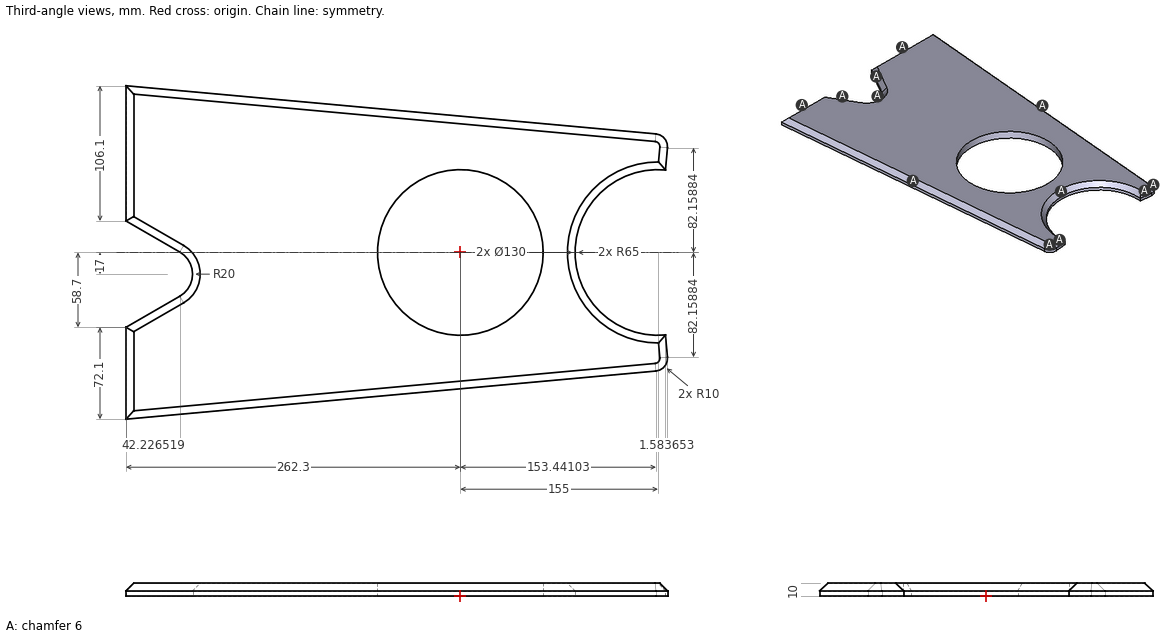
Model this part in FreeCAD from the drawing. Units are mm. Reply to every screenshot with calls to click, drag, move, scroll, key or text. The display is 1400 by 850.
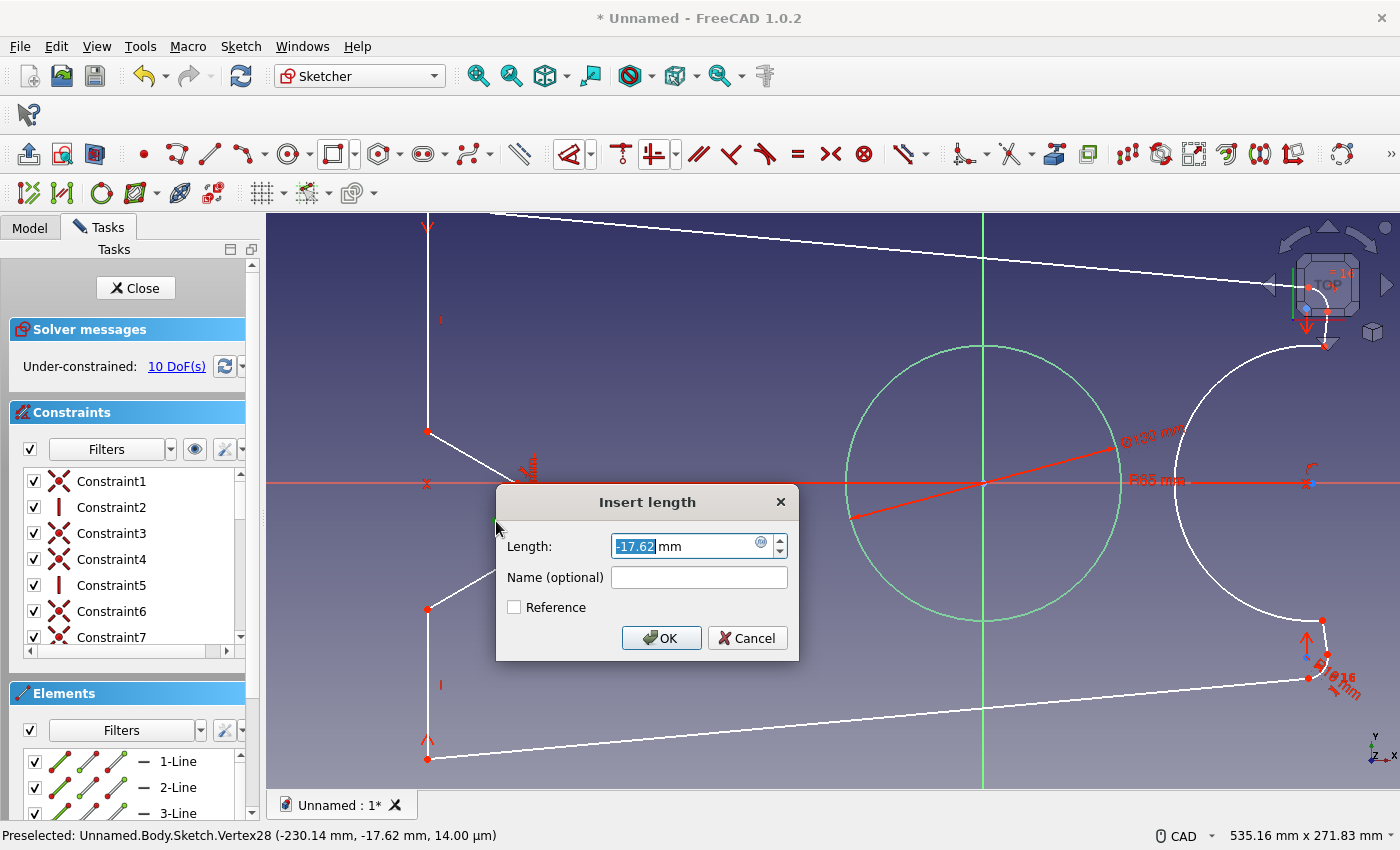
text(-17)
key(Return)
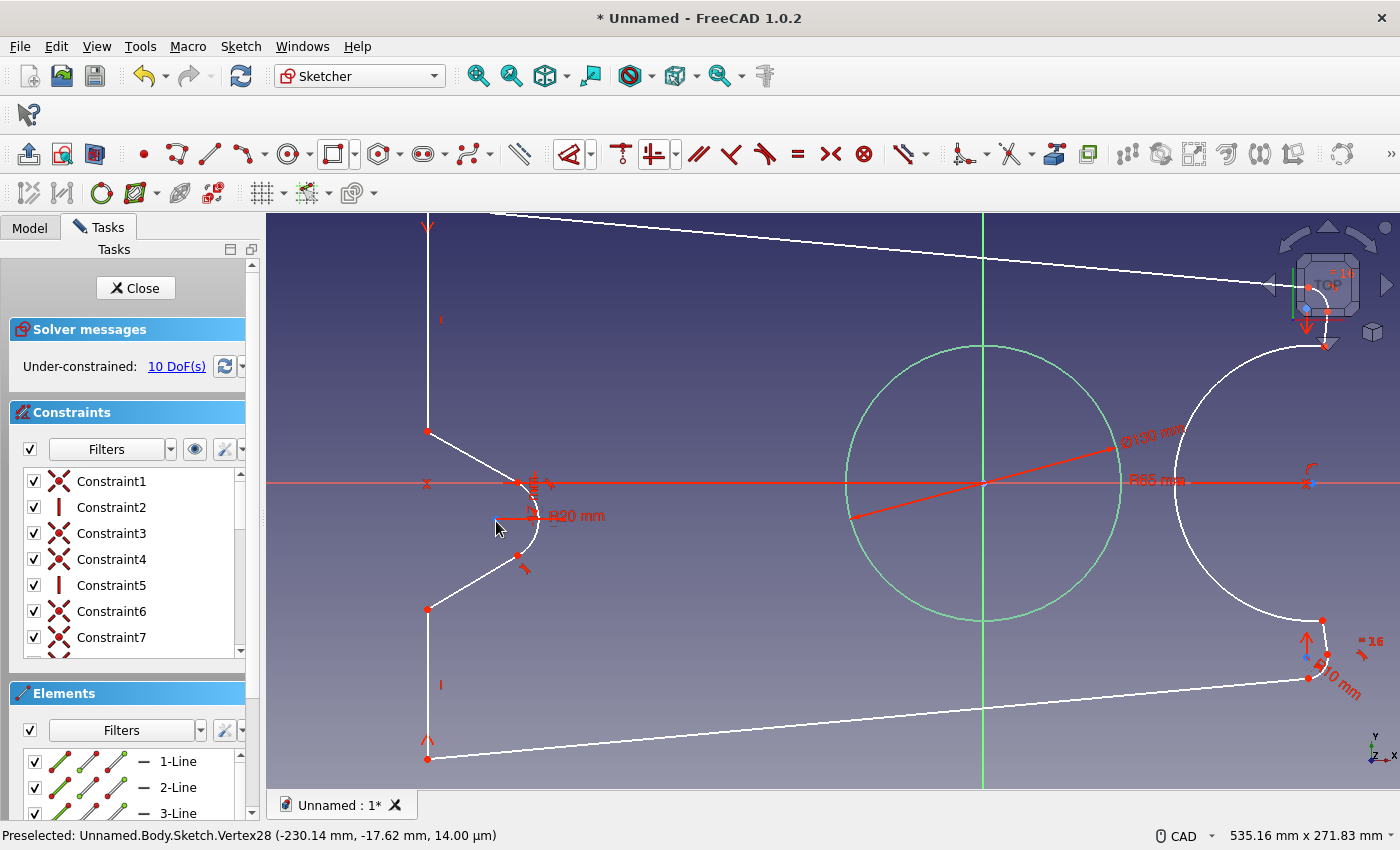
click(428, 654)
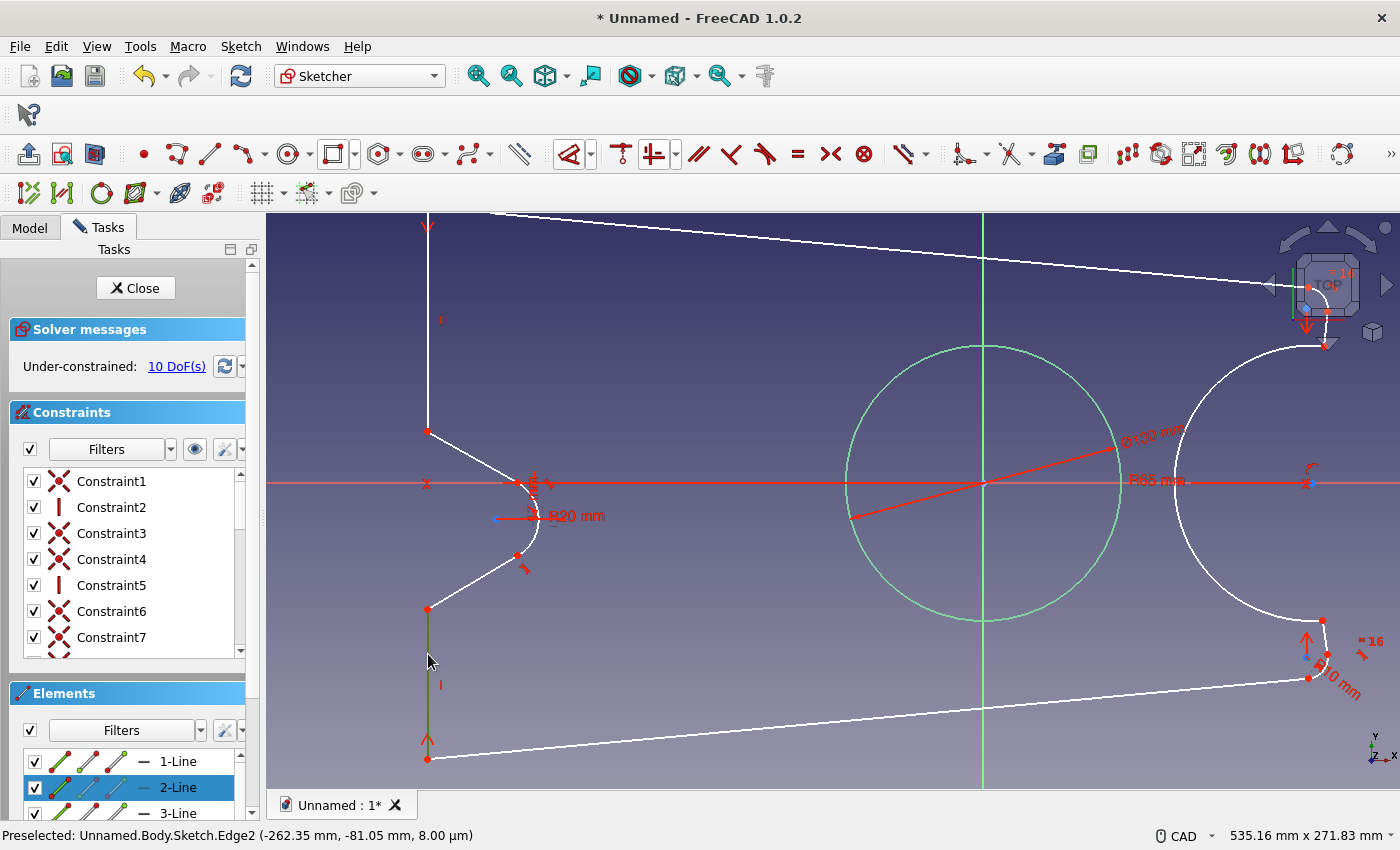
key(i)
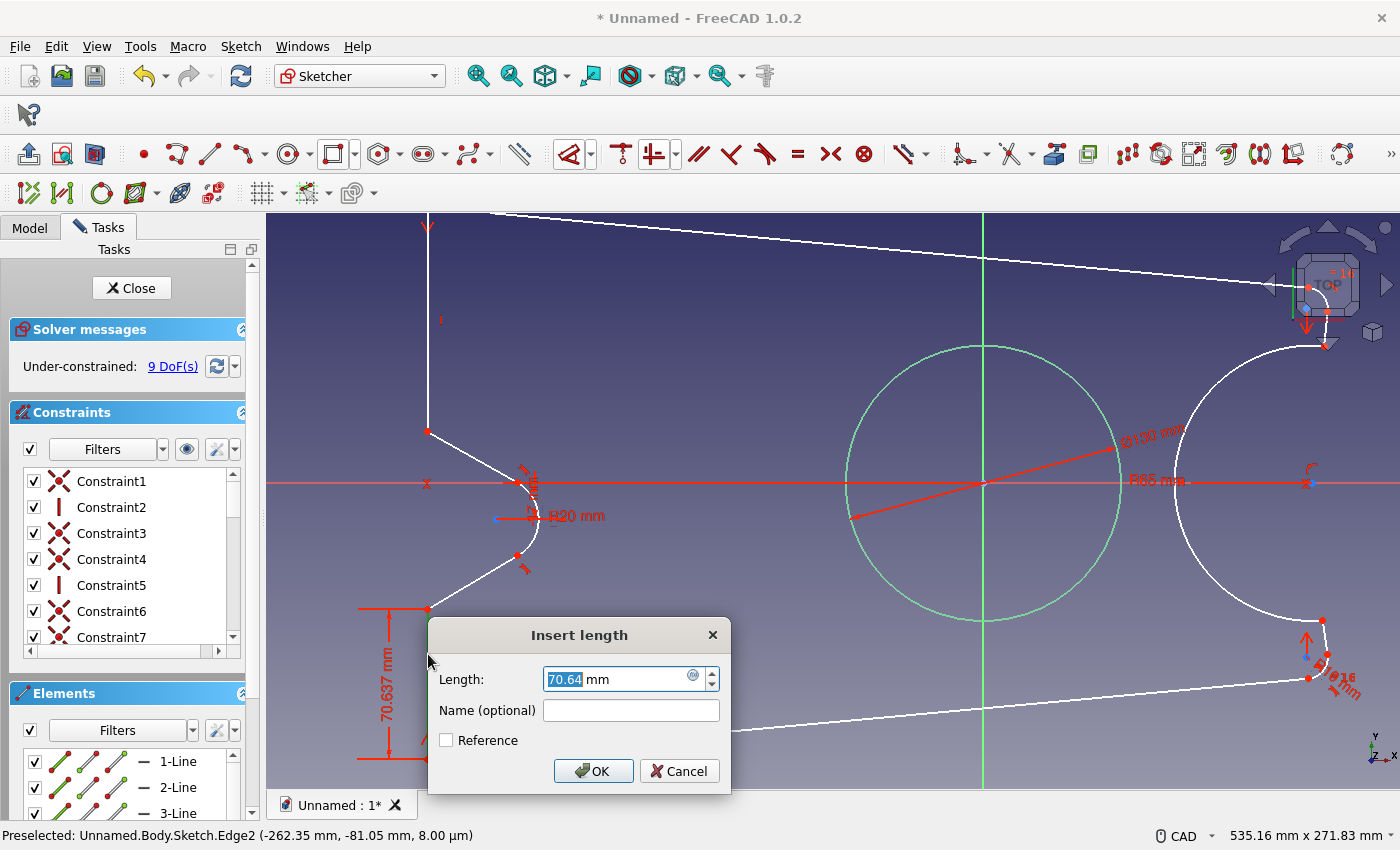
text(72.1)
key(Return)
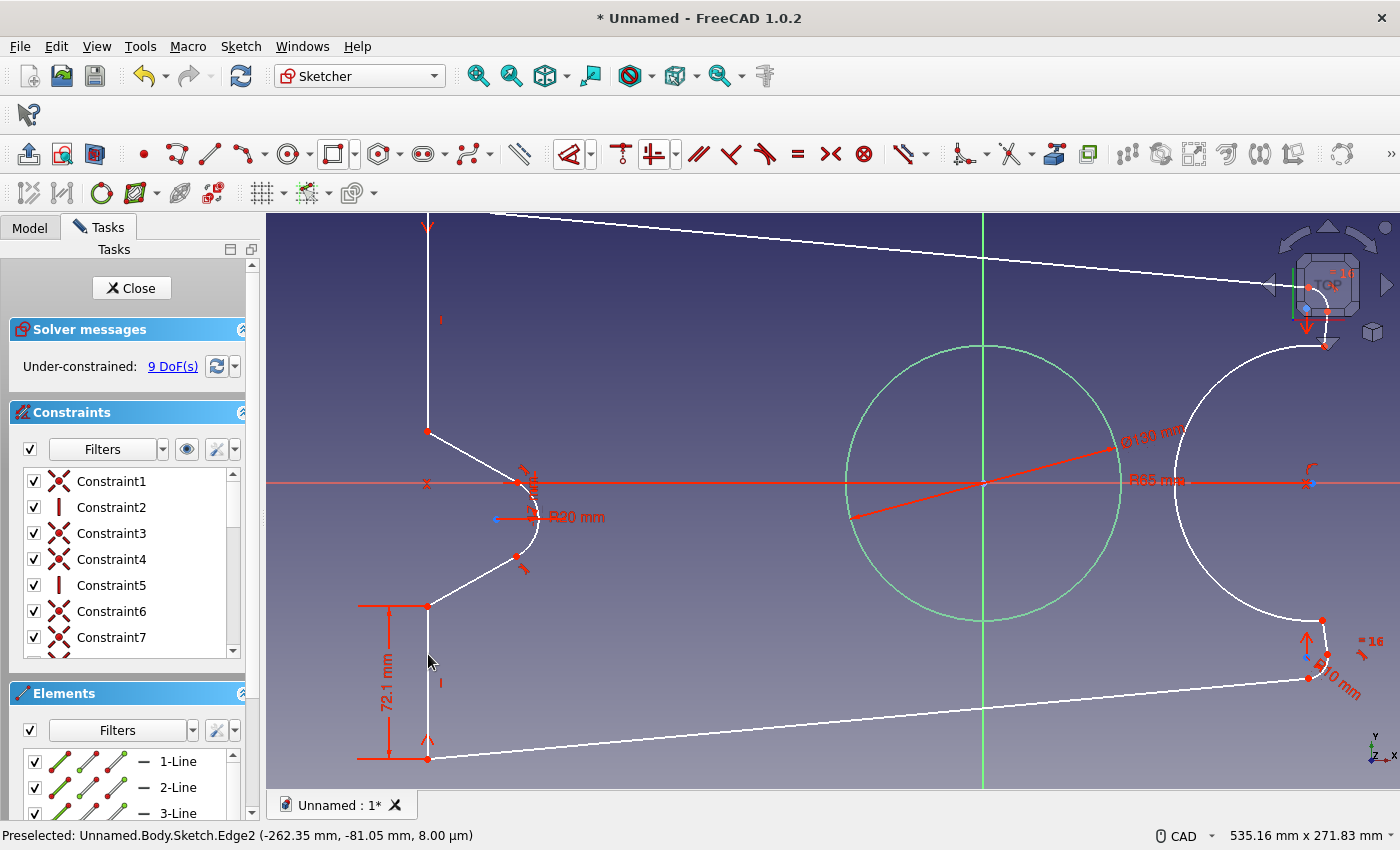
scroll(534, 537, down, 2)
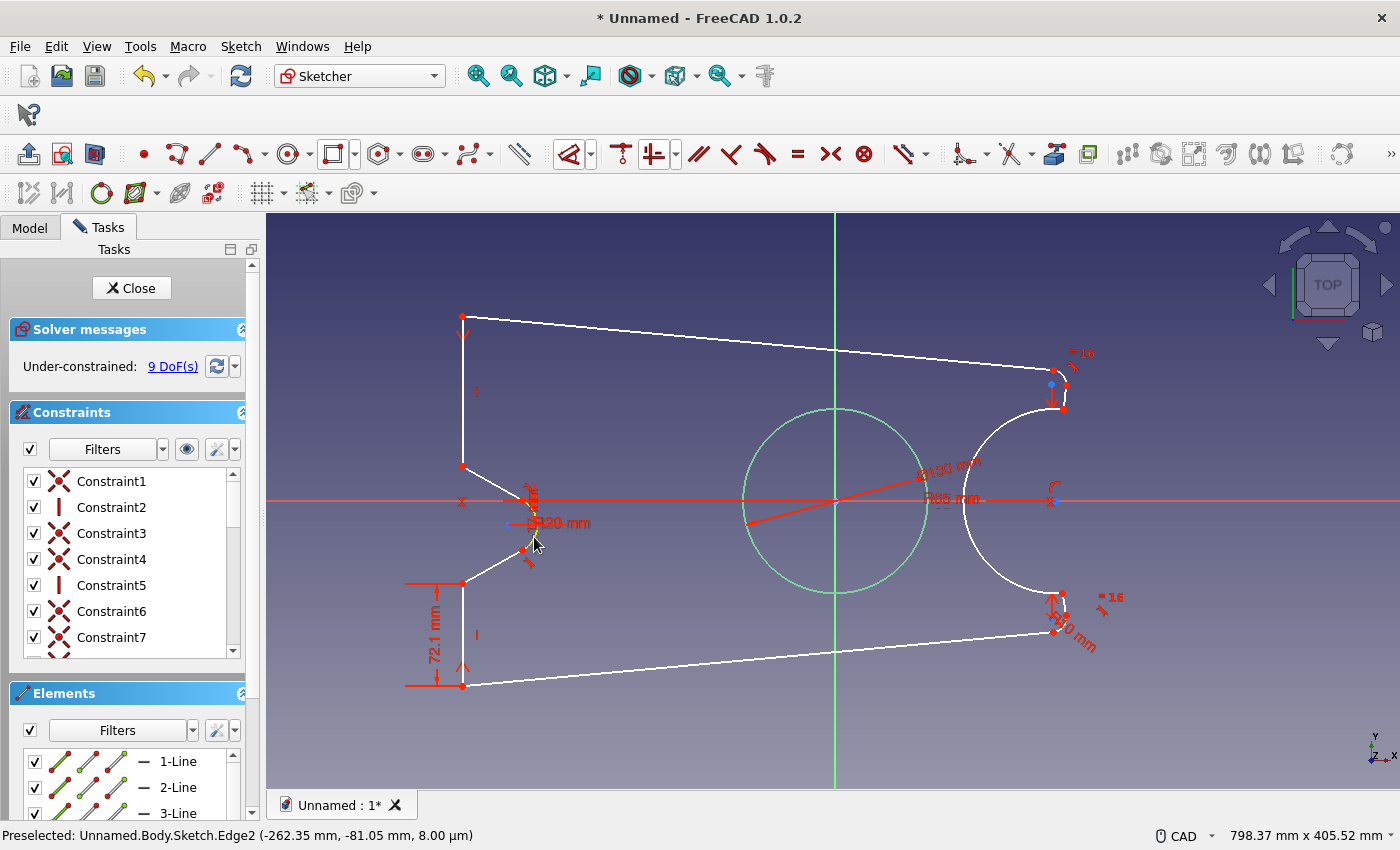
click(1056, 501)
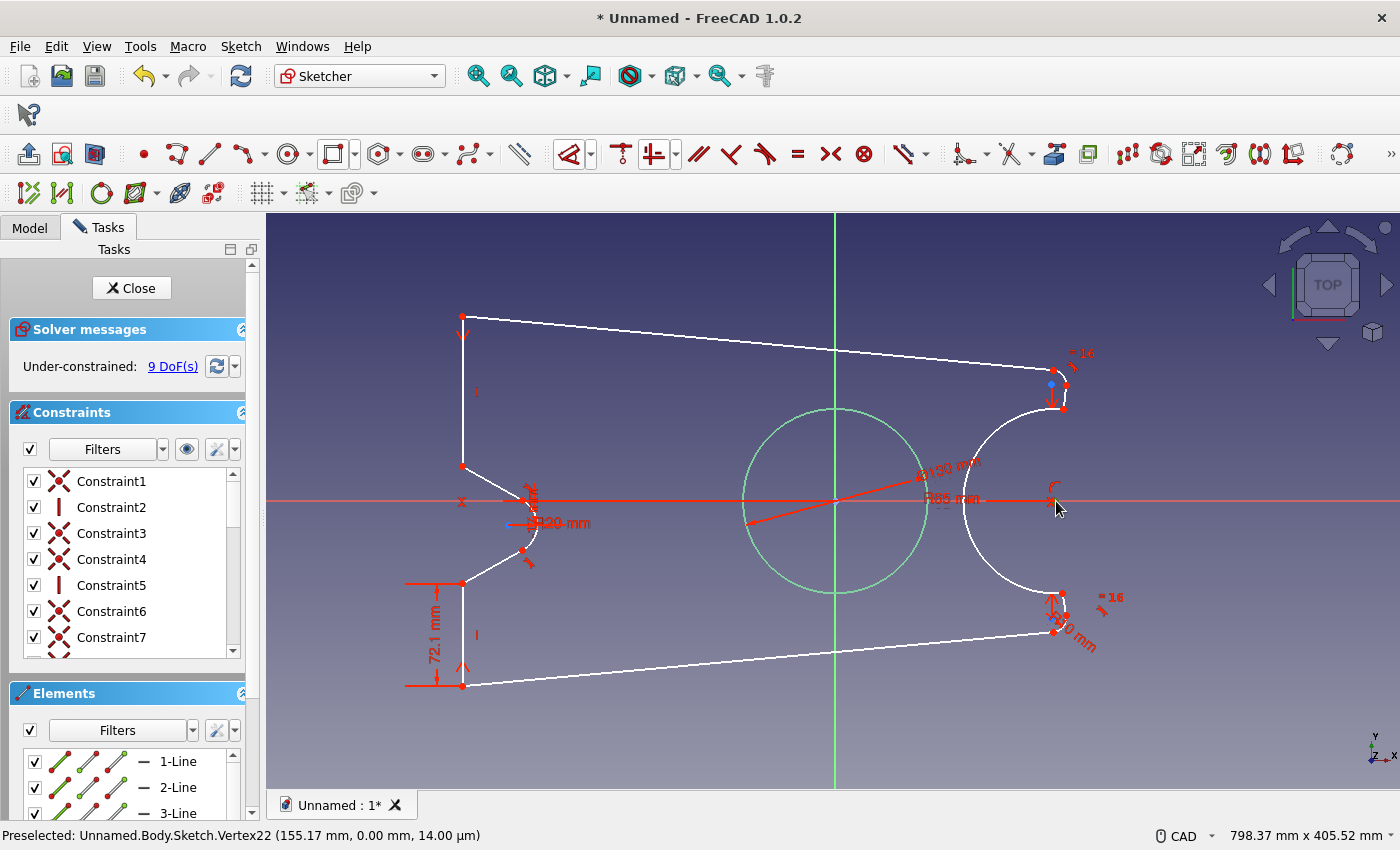
key(l)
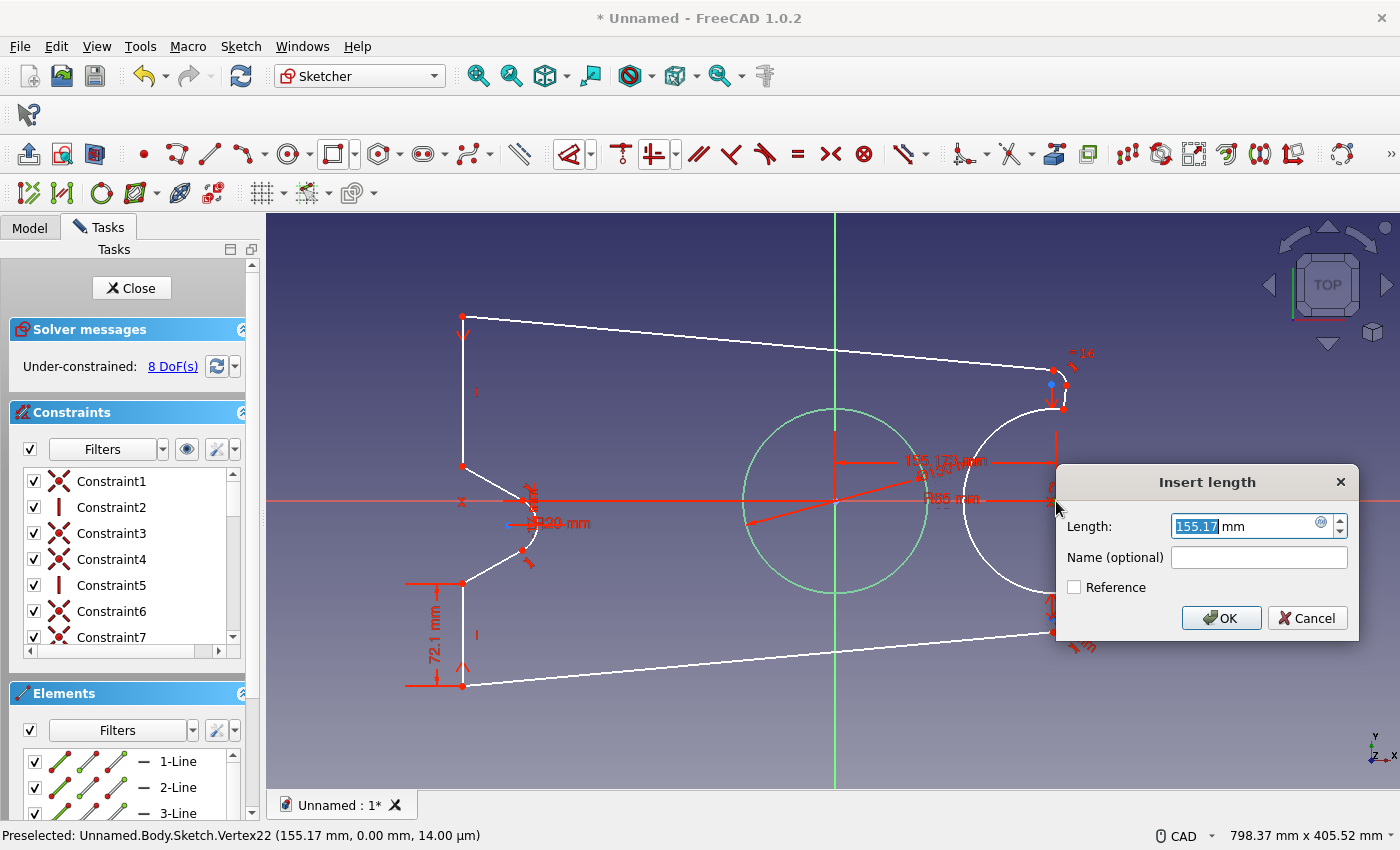
text(155)
key(Return)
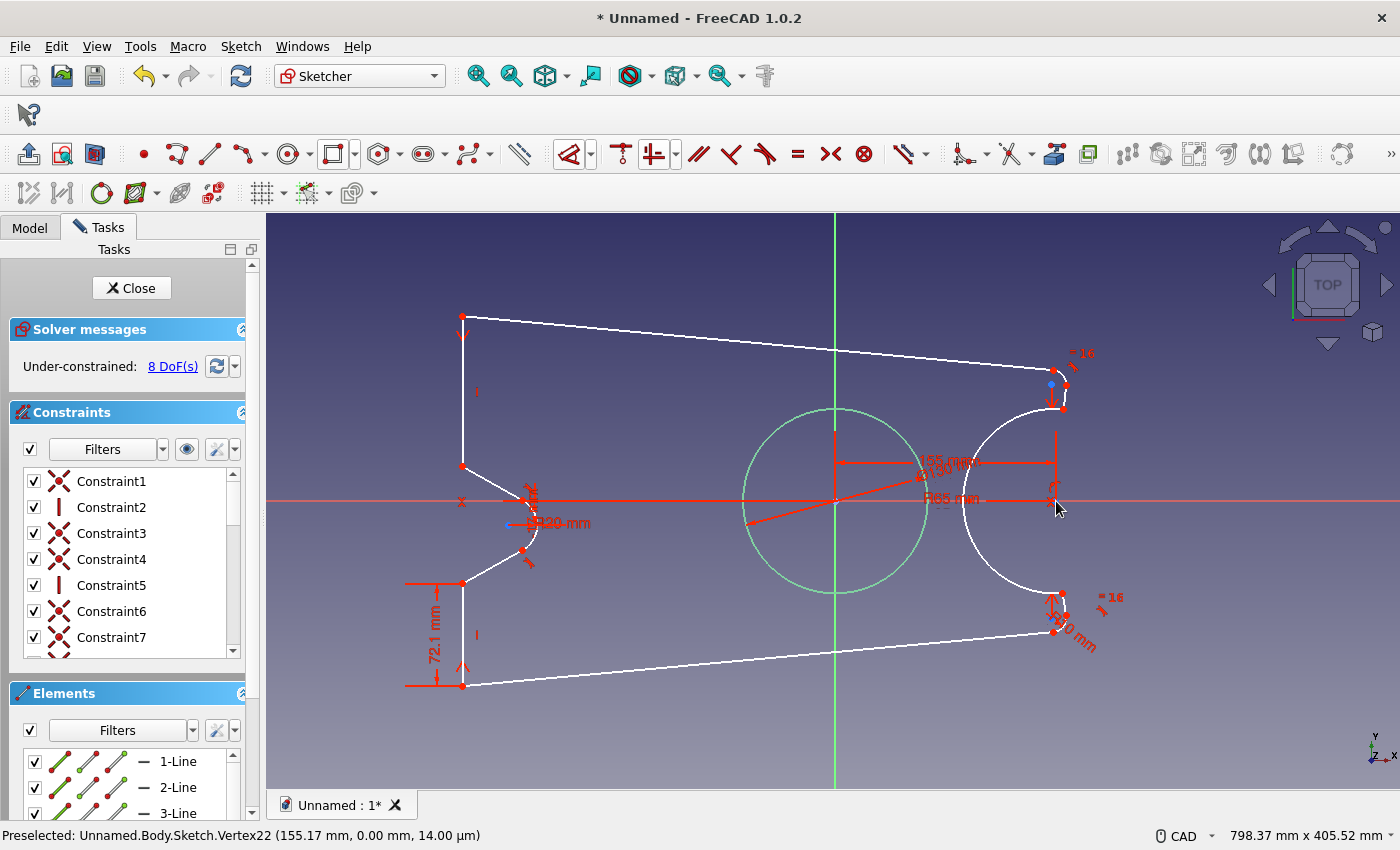
click(463, 361)